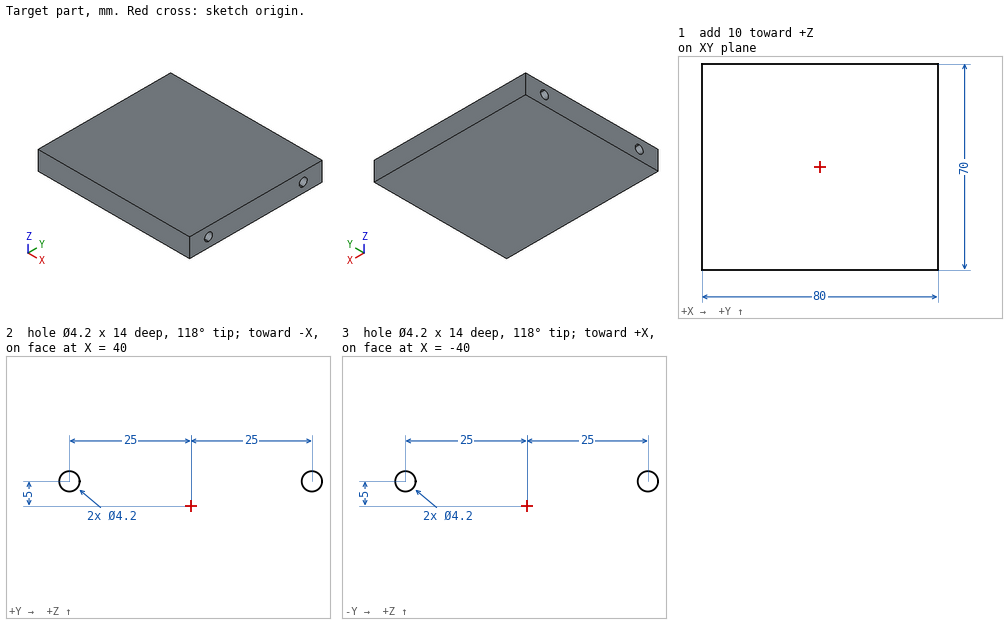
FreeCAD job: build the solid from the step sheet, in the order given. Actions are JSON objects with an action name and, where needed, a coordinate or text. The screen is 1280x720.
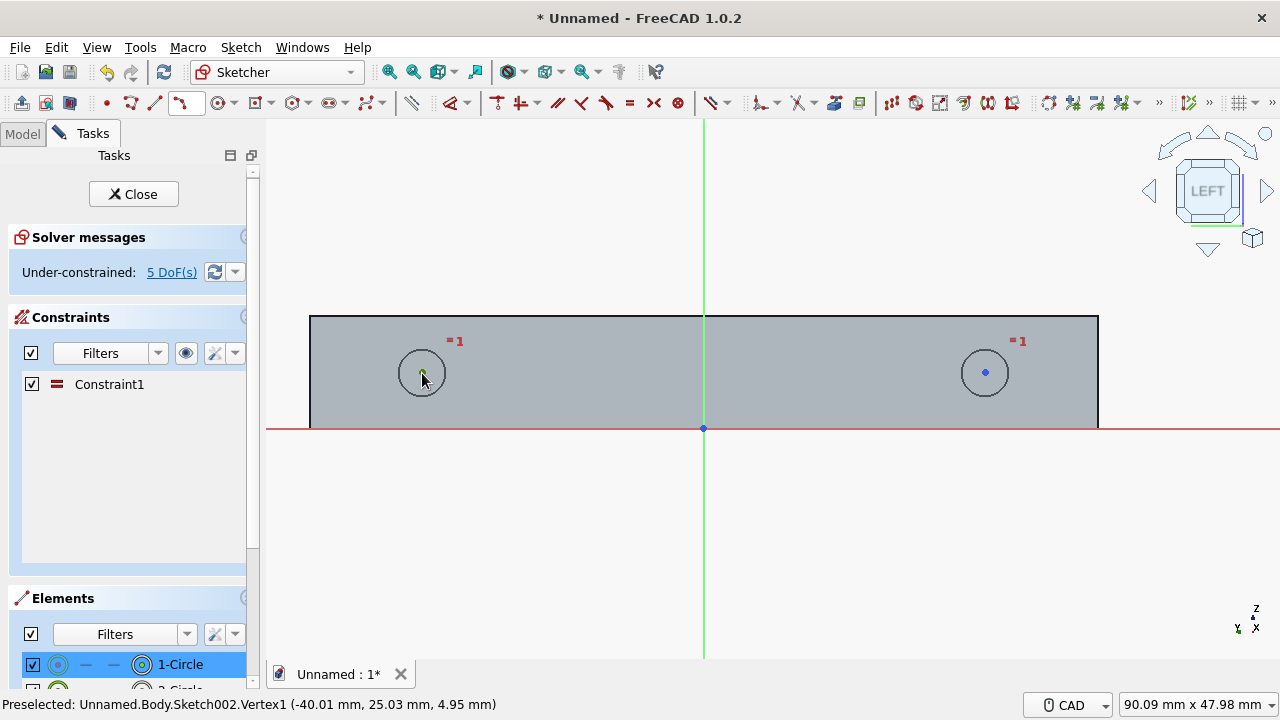
{"action": "left_click", "coordinate": [985, 373]}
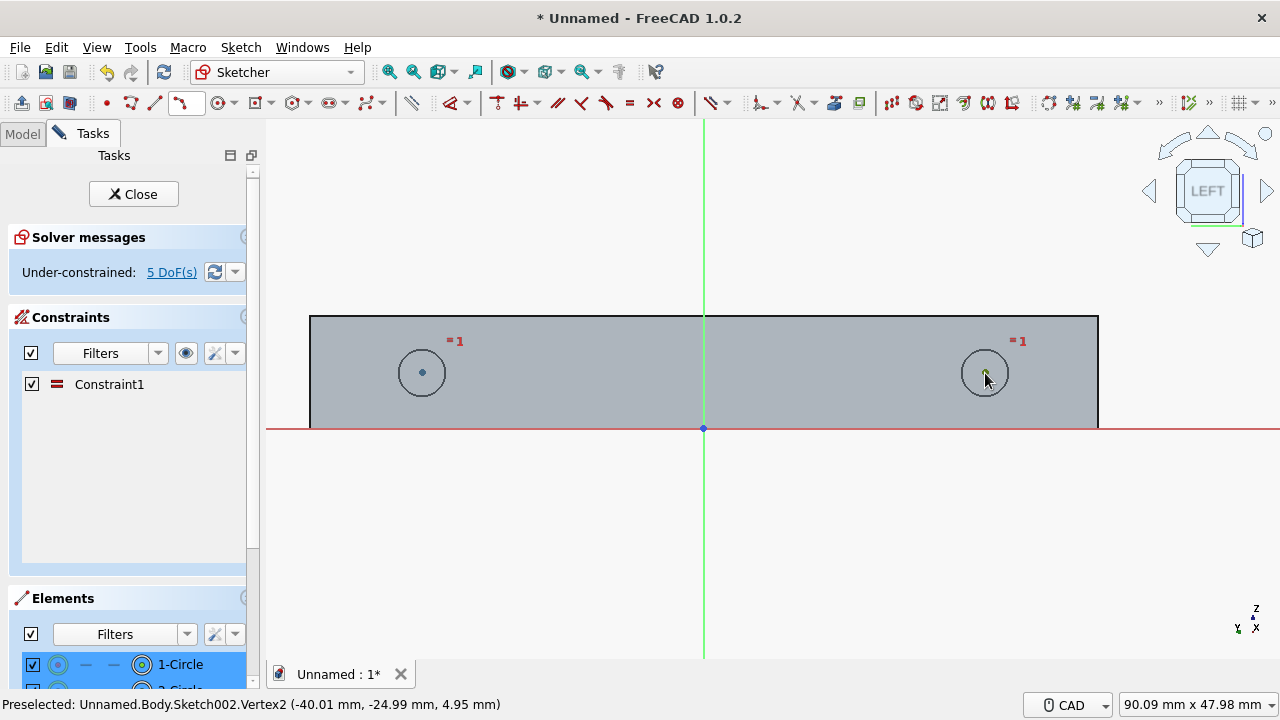
{"action": "key", "text": "h"}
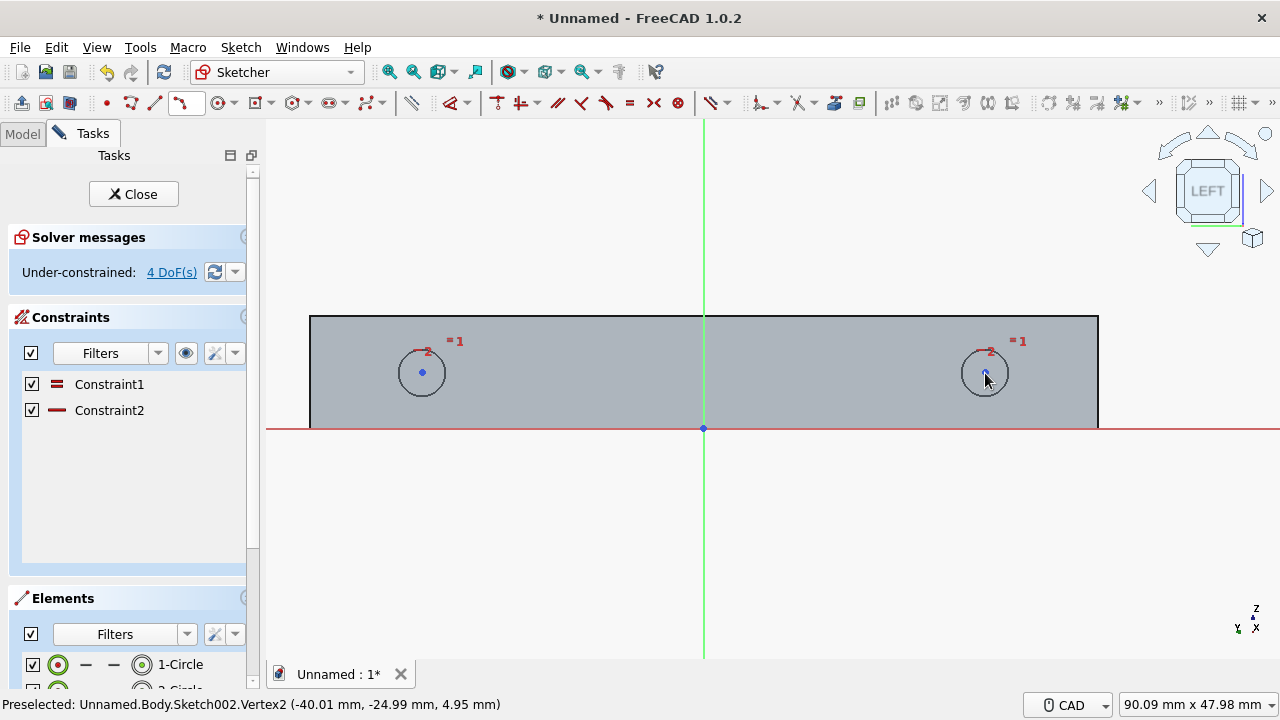
{"action": "left_click", "coordinate": [450, 104]}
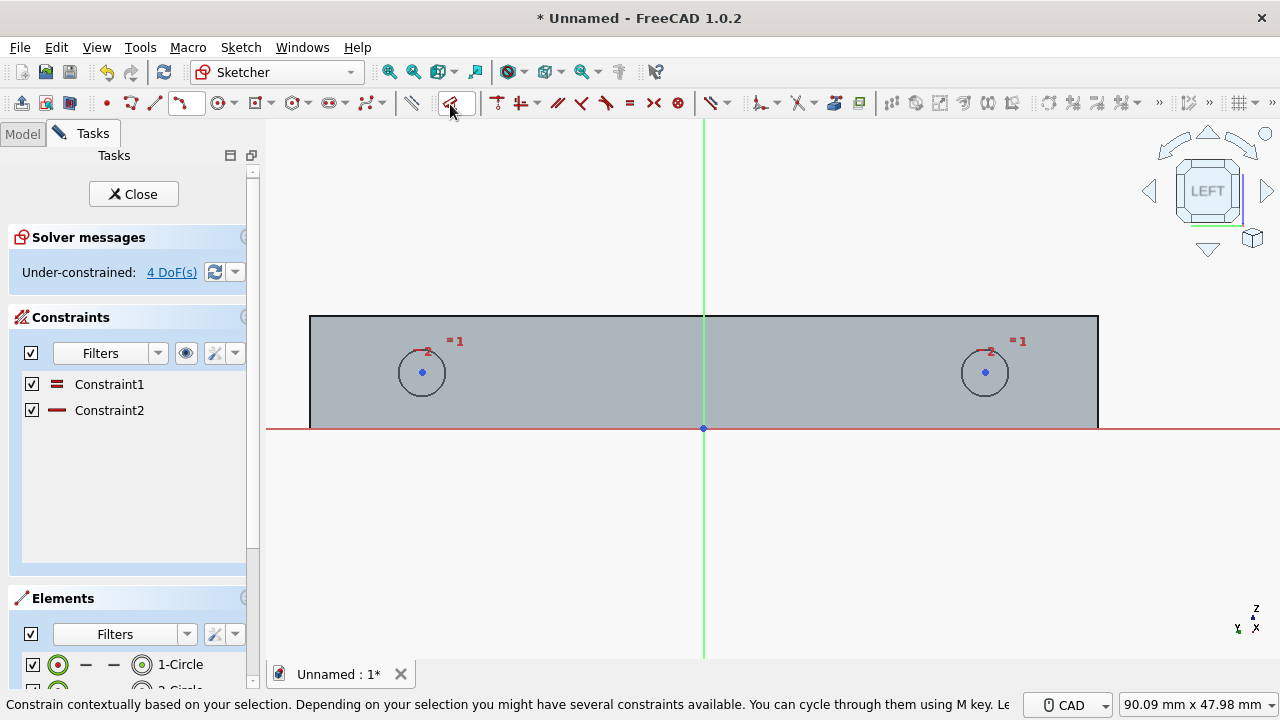
{"action": "left_click", "coordinate": [438, 356]}
{"action": "left_click", "coordinate": [460, 333]}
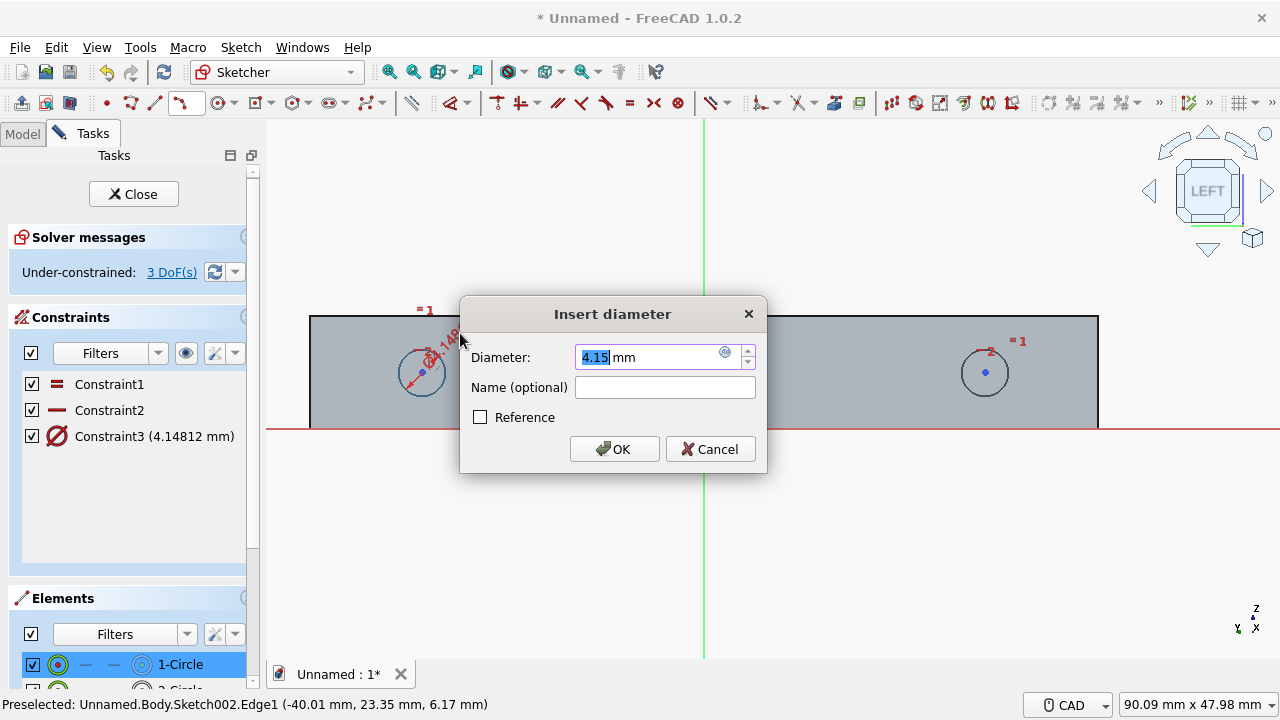
{"action": "type", "text": "4.2"}
{"action": "key", "text": "Return"}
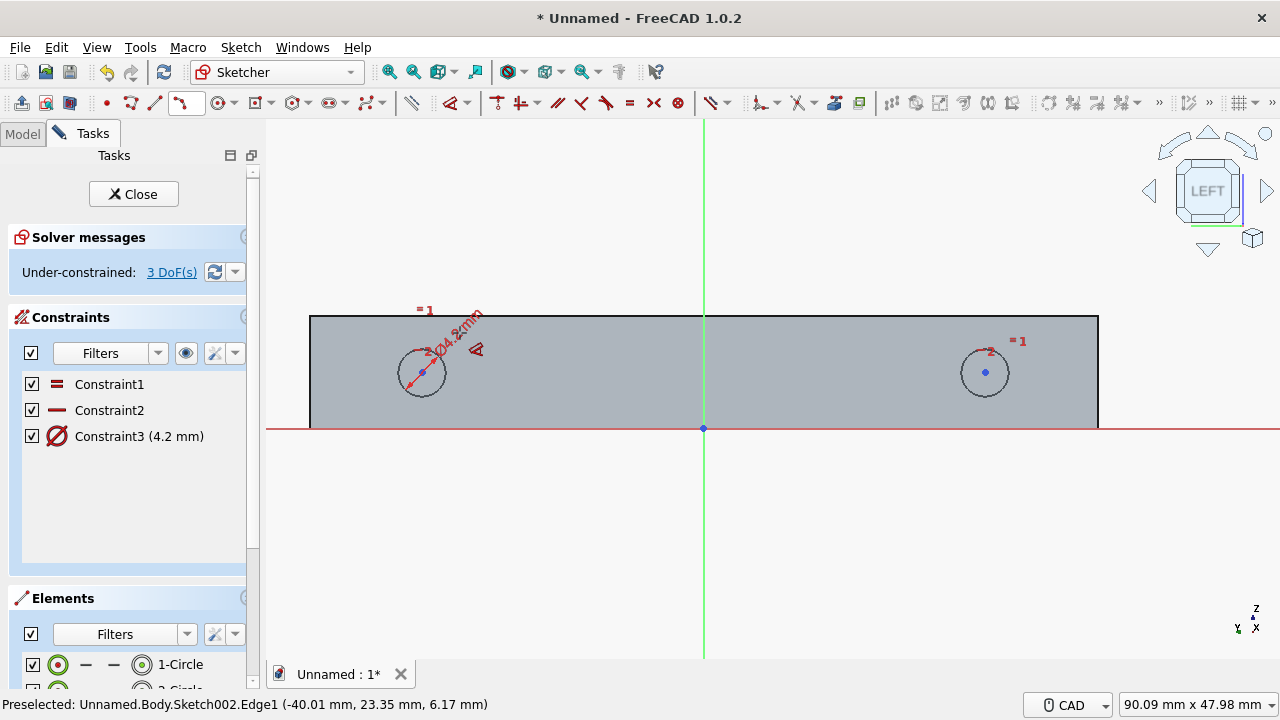
{"action": "left_click", "coordinate": [422, 373]}
{"action": "left_click", "coordinate": [388, 401]}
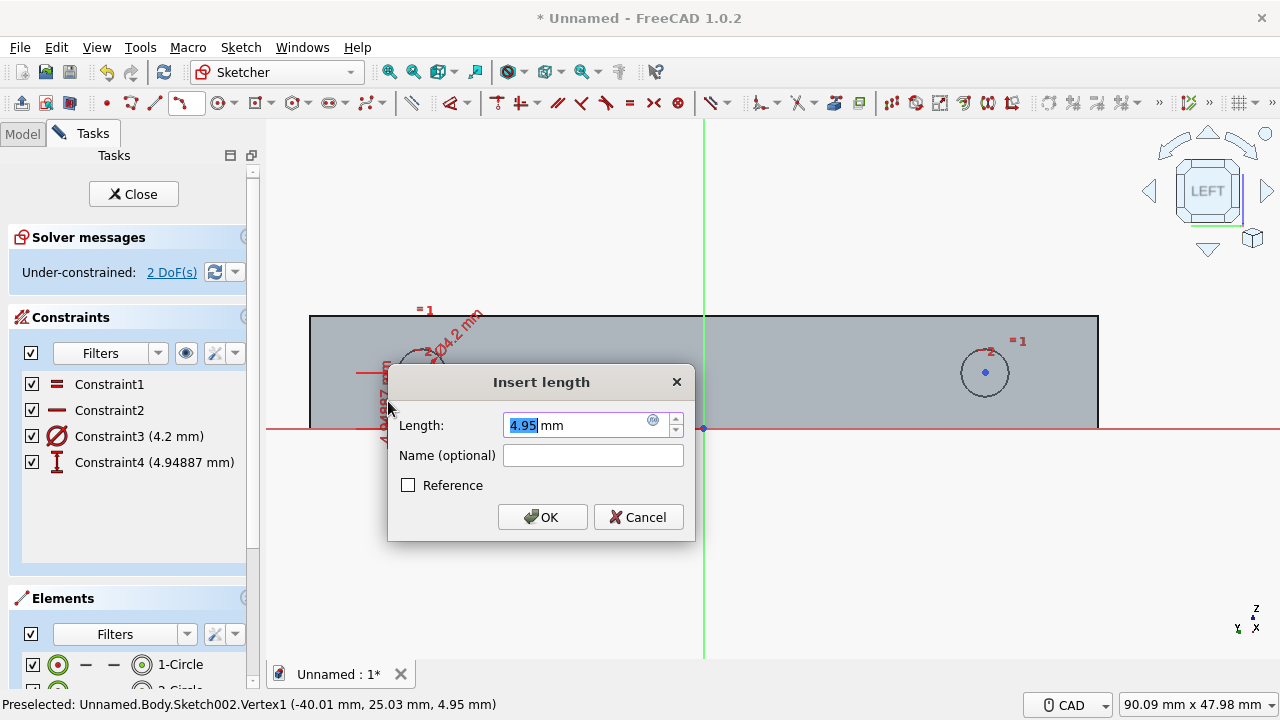
{"action": "type", "text": "5"}
{"action": "key", "text": "Return"}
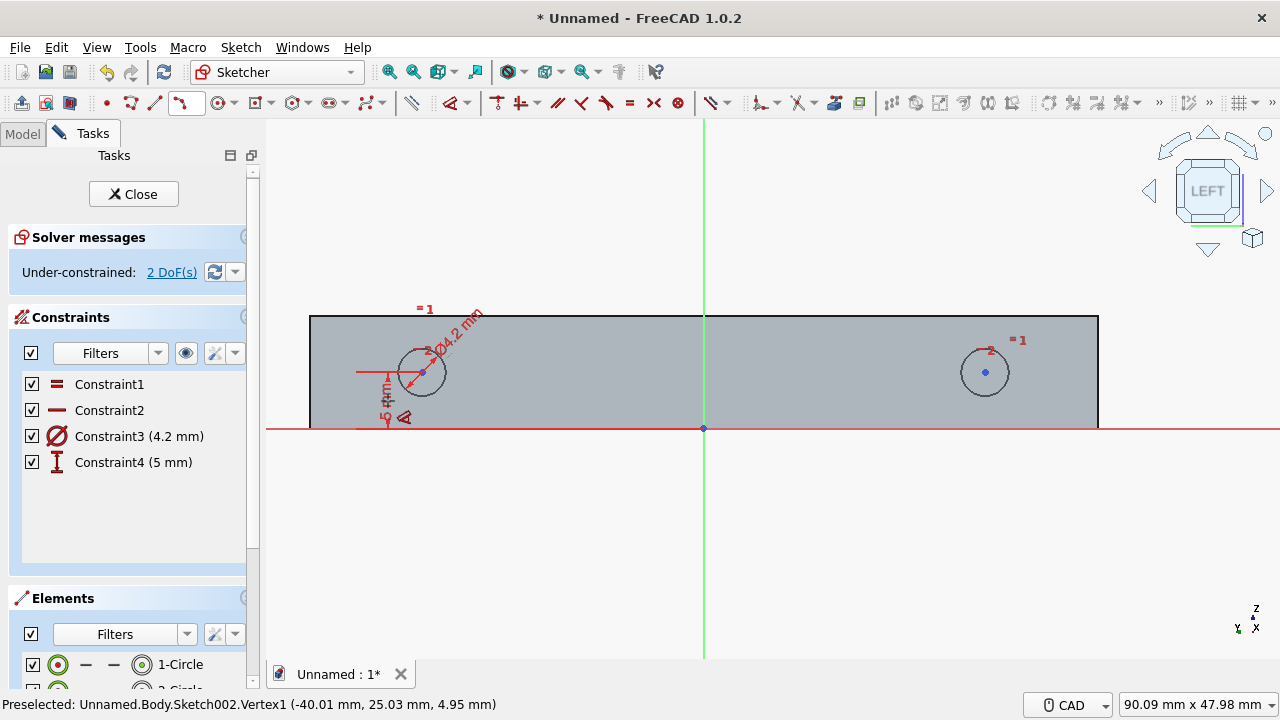
{"action": "left_click", "coordinate": [422, 372]}
{"action": "left_click", "coordinate": [563, 463]}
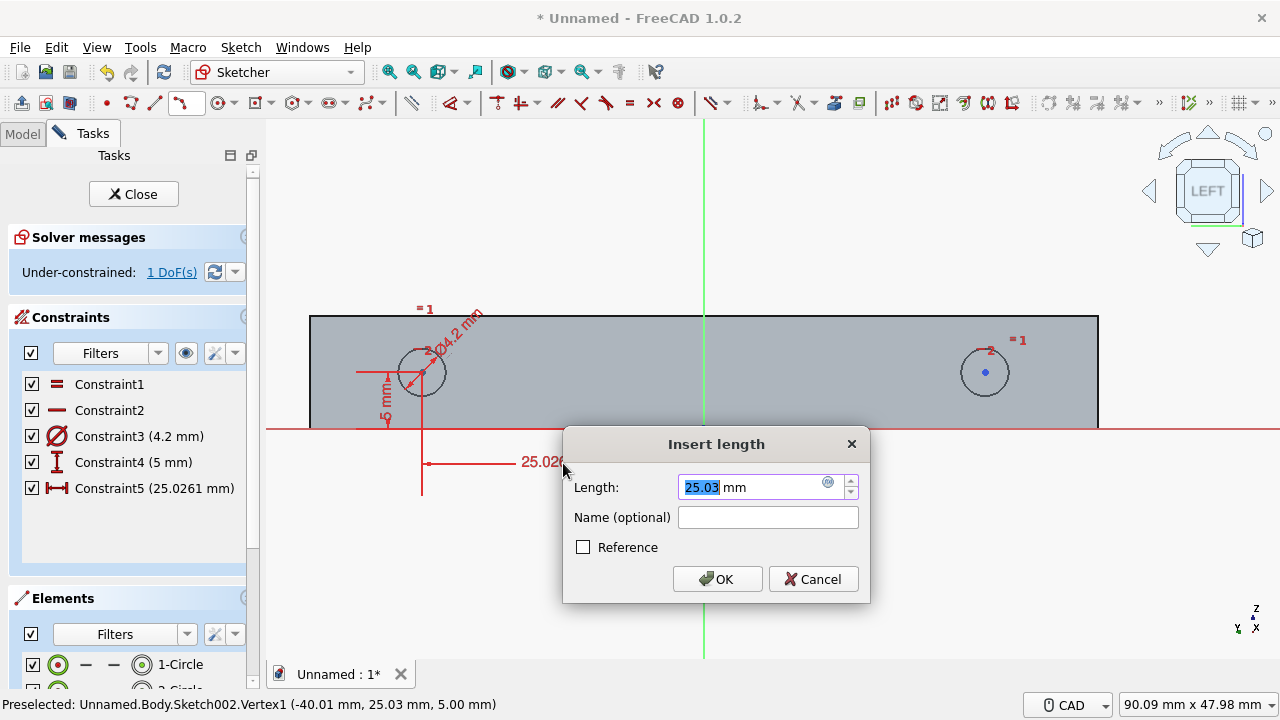
{"action": "type", "text": "25"}
{"action": "key", "text": "Return"}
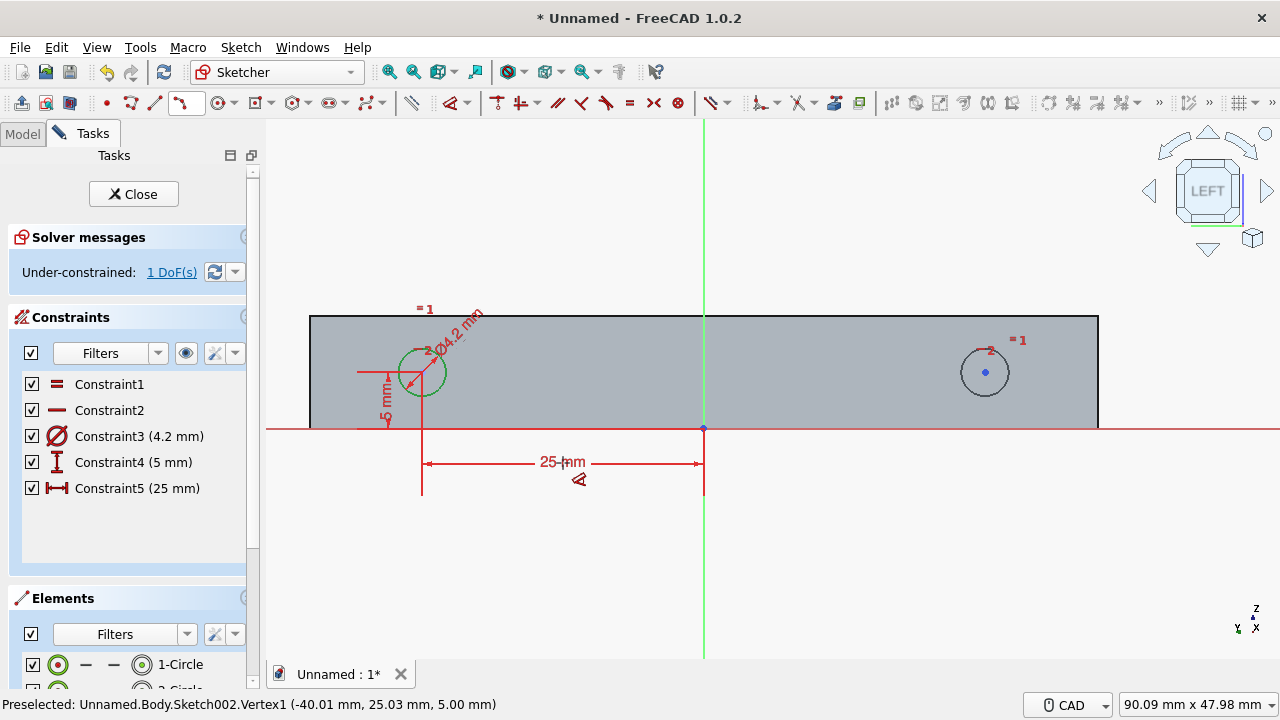
{"action": "left_click", "coordinate": [985, 372]}
{"action": "left_click", "coordinate": [844, 463]}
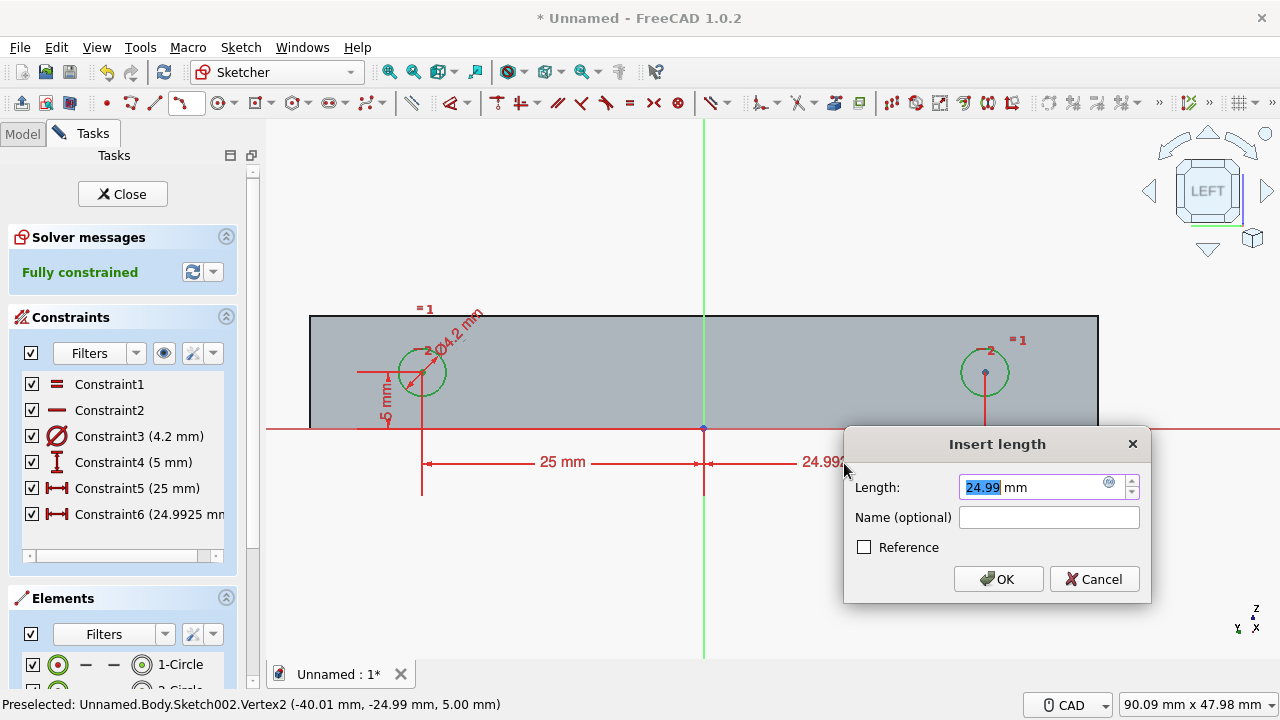
{"action": "type", "text": "25"}
{"action": "key", "text": "Return"}
{"action": "key", "text": "Escape"}